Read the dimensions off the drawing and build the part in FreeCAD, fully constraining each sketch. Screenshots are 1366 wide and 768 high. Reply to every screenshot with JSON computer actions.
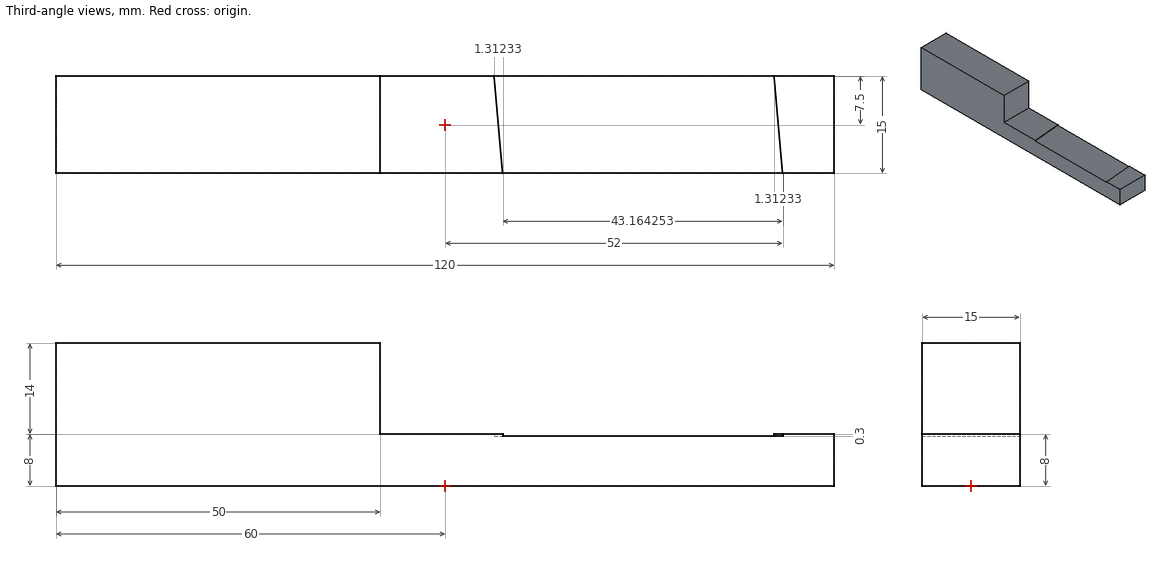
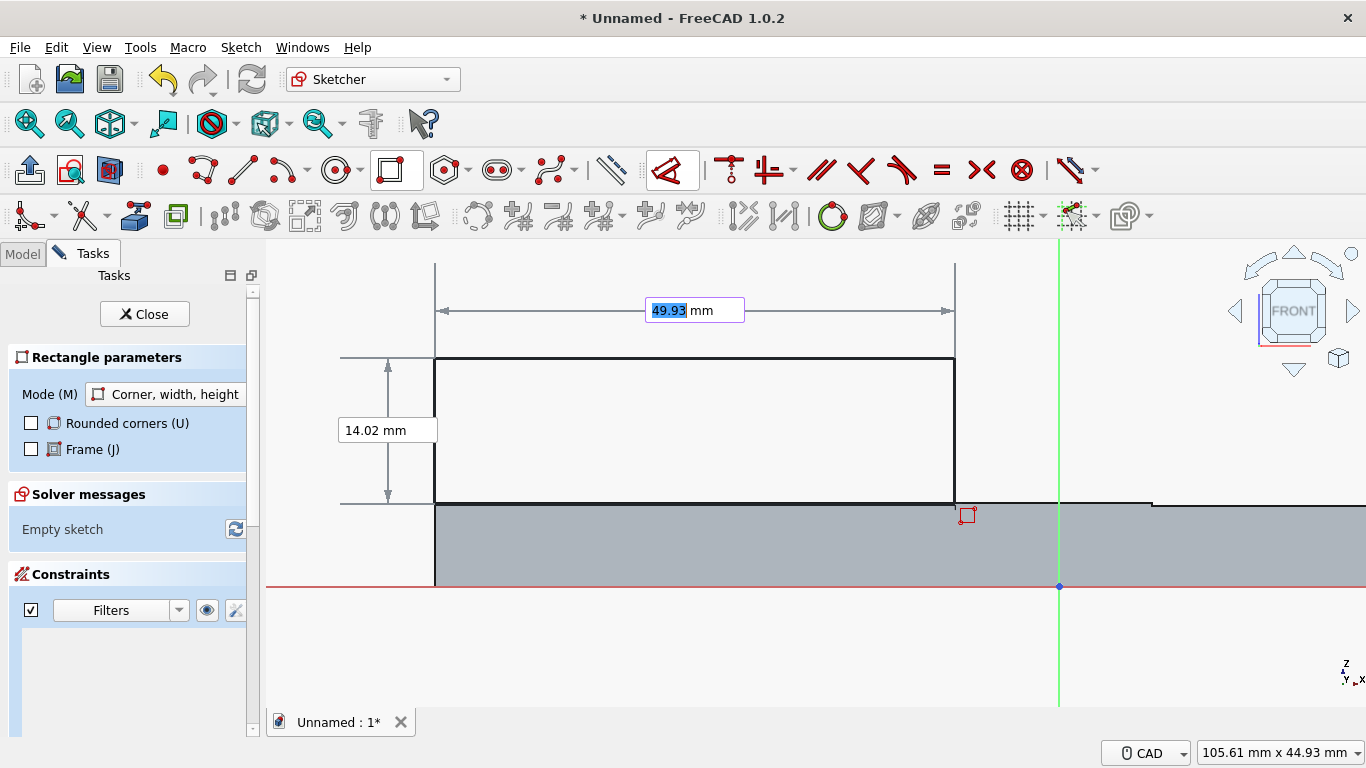
{"action": "type", "text": "50"}
{"action": "key", "text": "Tab"}
{"action": "type", "text": "14"}
{"action": "key", "text": "Return"}
{"action": "key", "text": "Escape"}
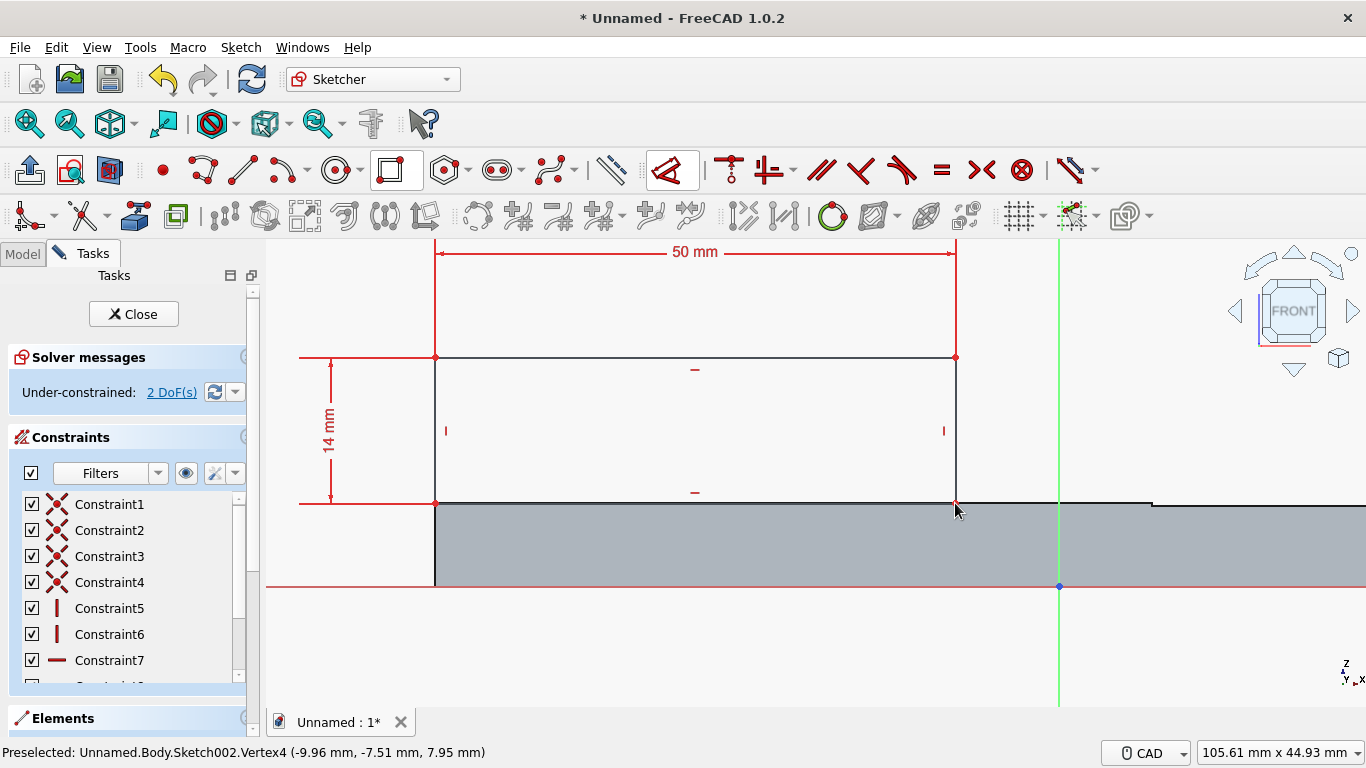
{"action": "left_click", "coordinate": [435, 504]}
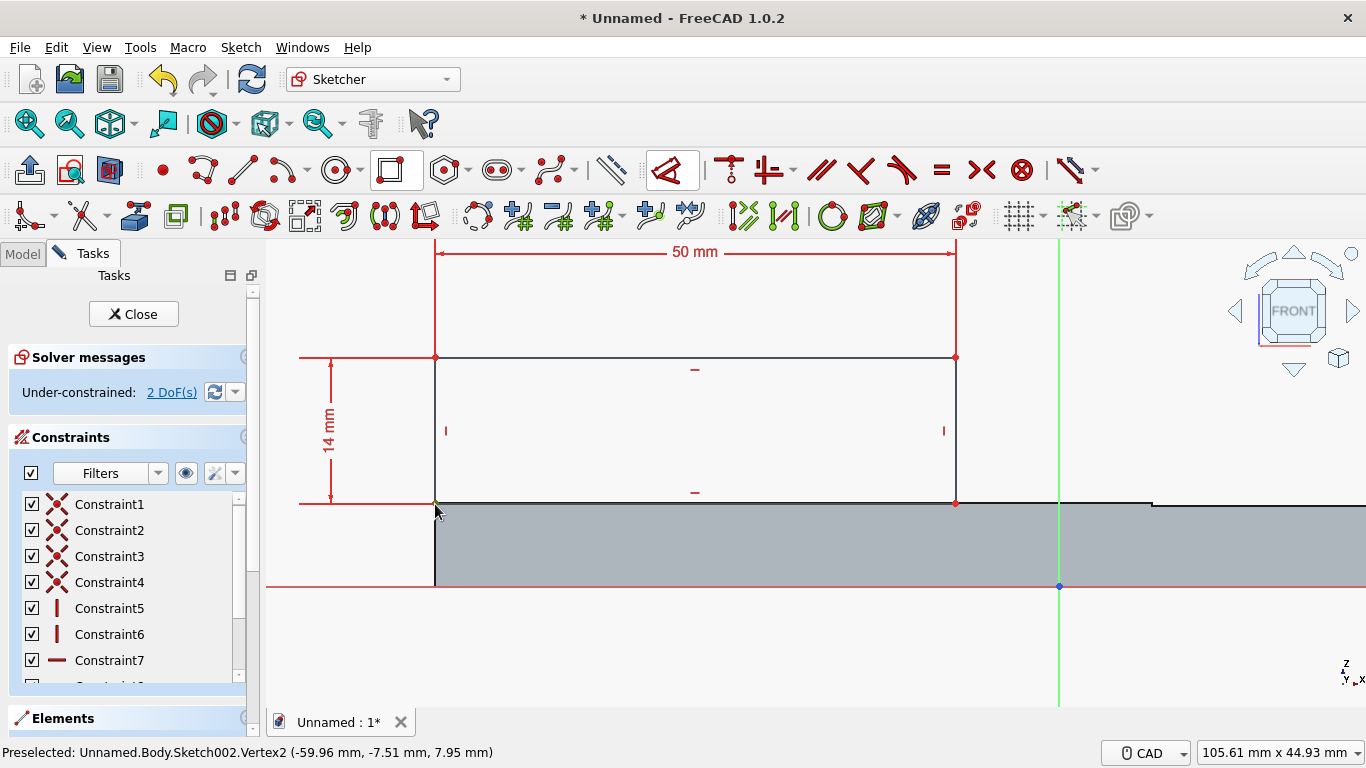
{"action": "key", "text": "i"}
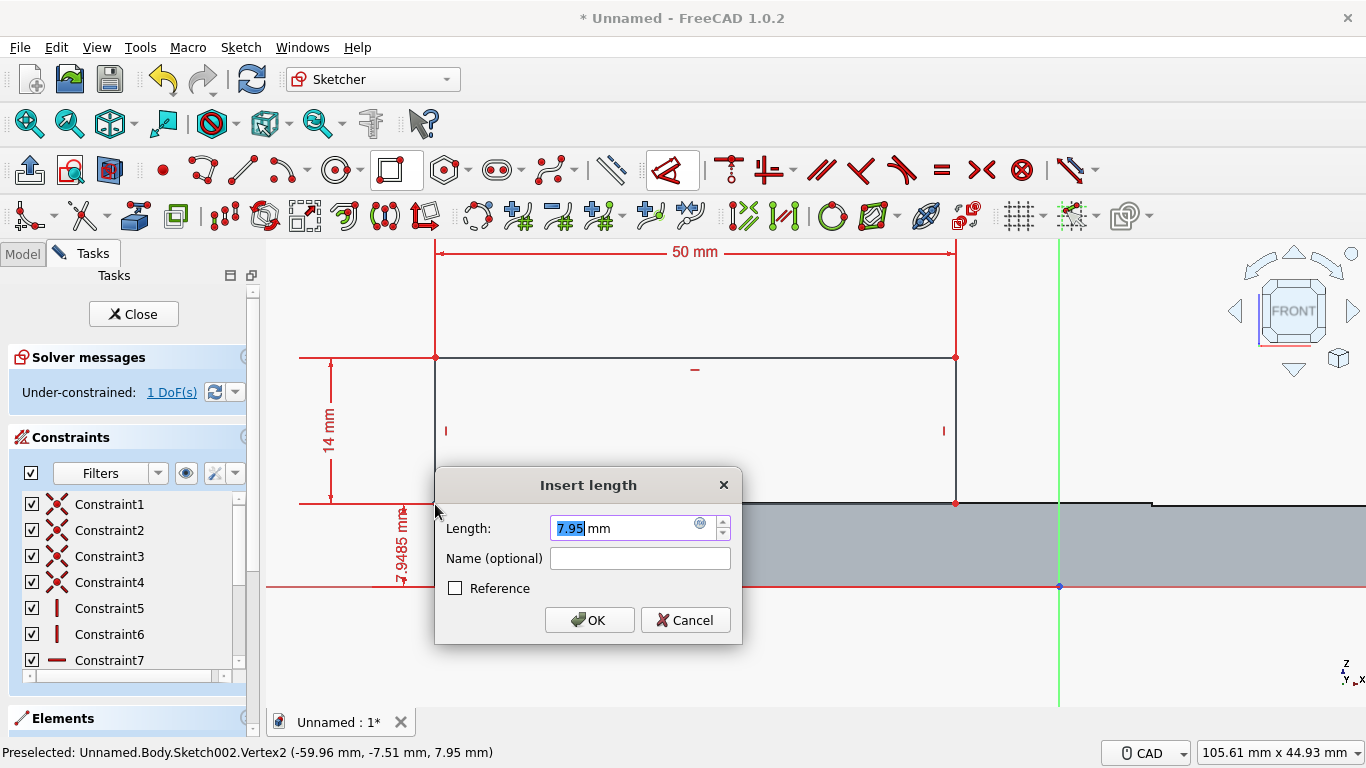
{"action": "type", "text": "8"}
{"action": "key", "text": "Return"}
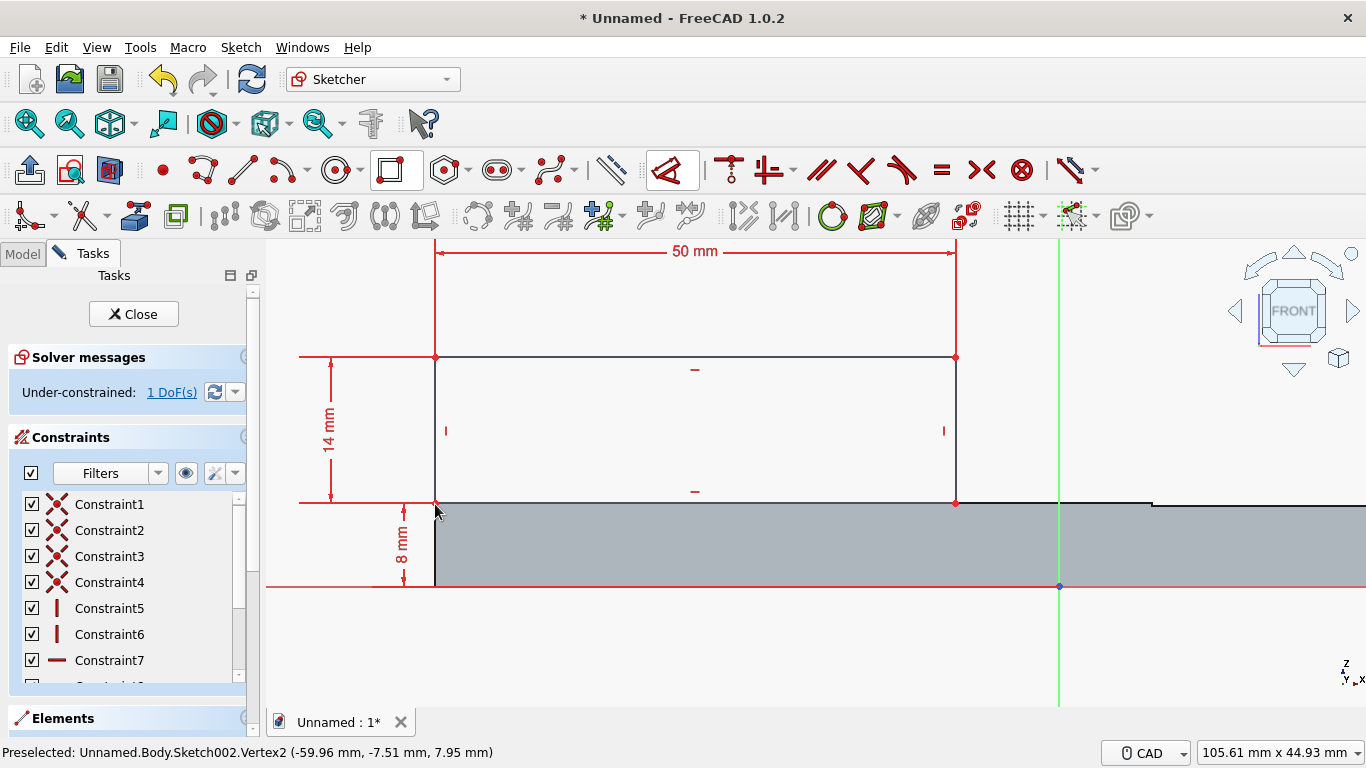
{"action": "left_click", "coordinate": [435, 357]}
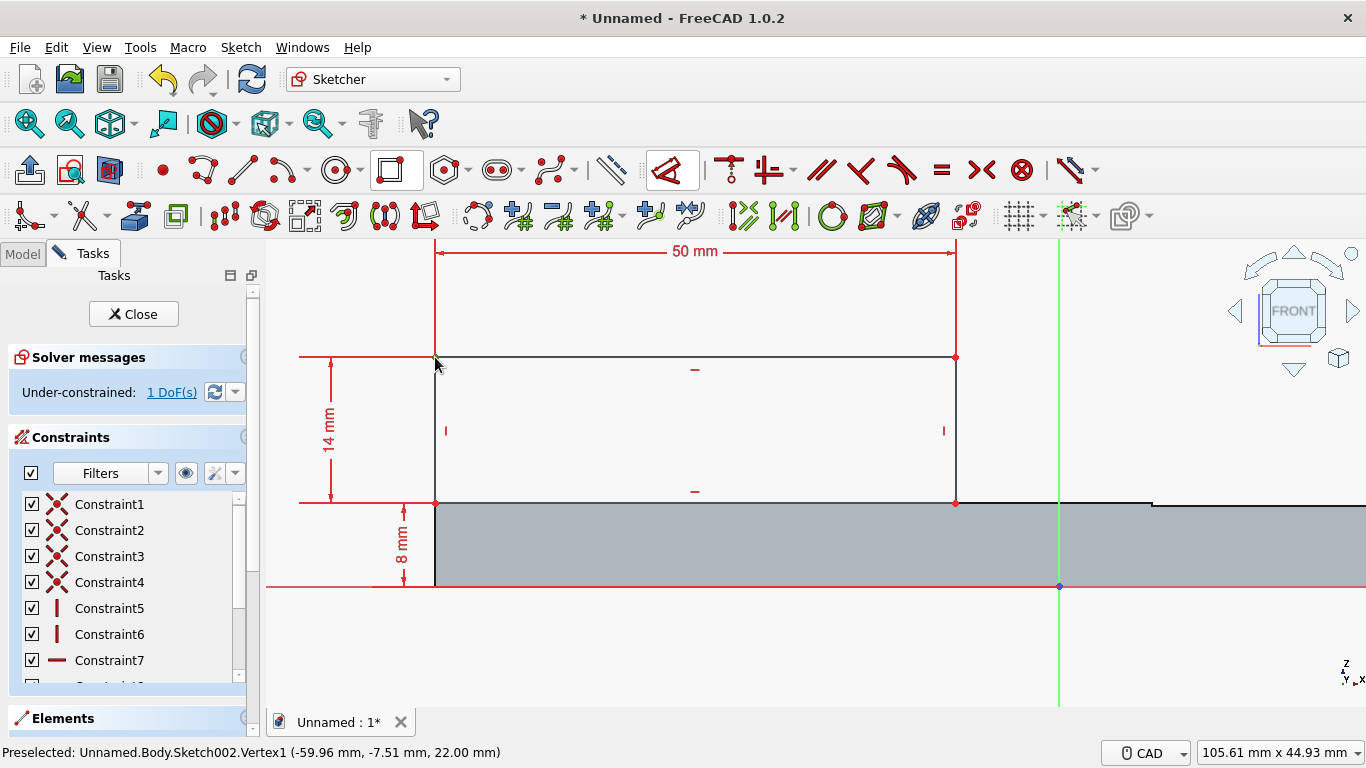
{"action": "left_click", "coordinate": [694, 170]}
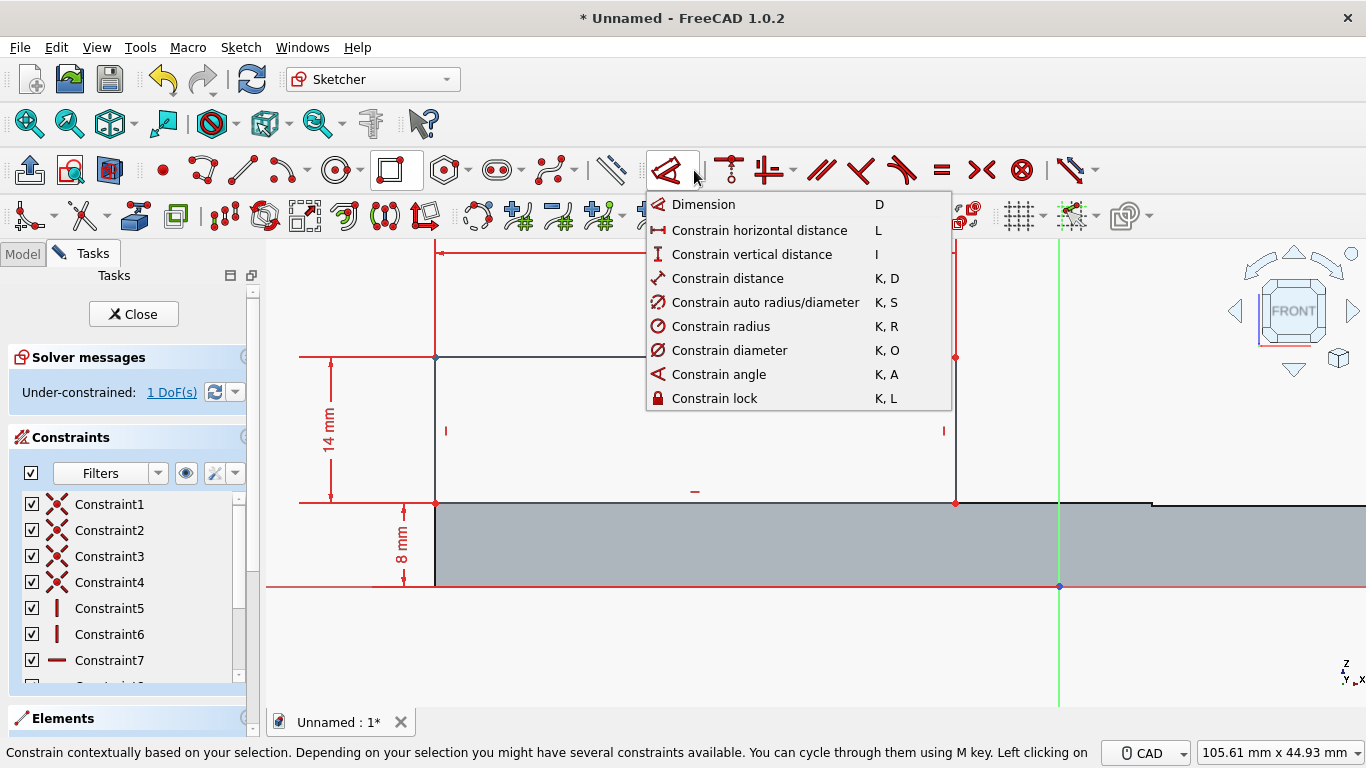
{"action": "left_click", "coordinate": [799, 230]}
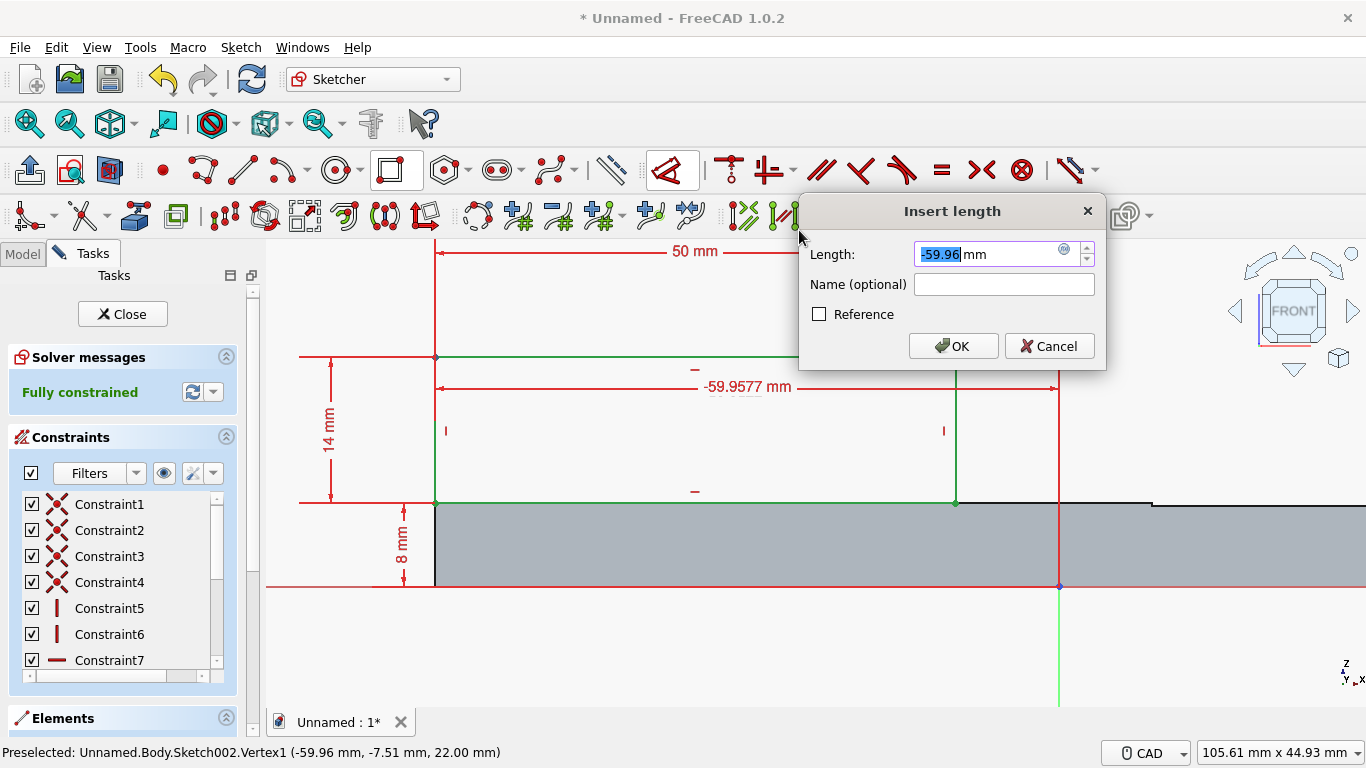
{"action": "type", "text": "-60"}
{"action": "key", "text": "Return"}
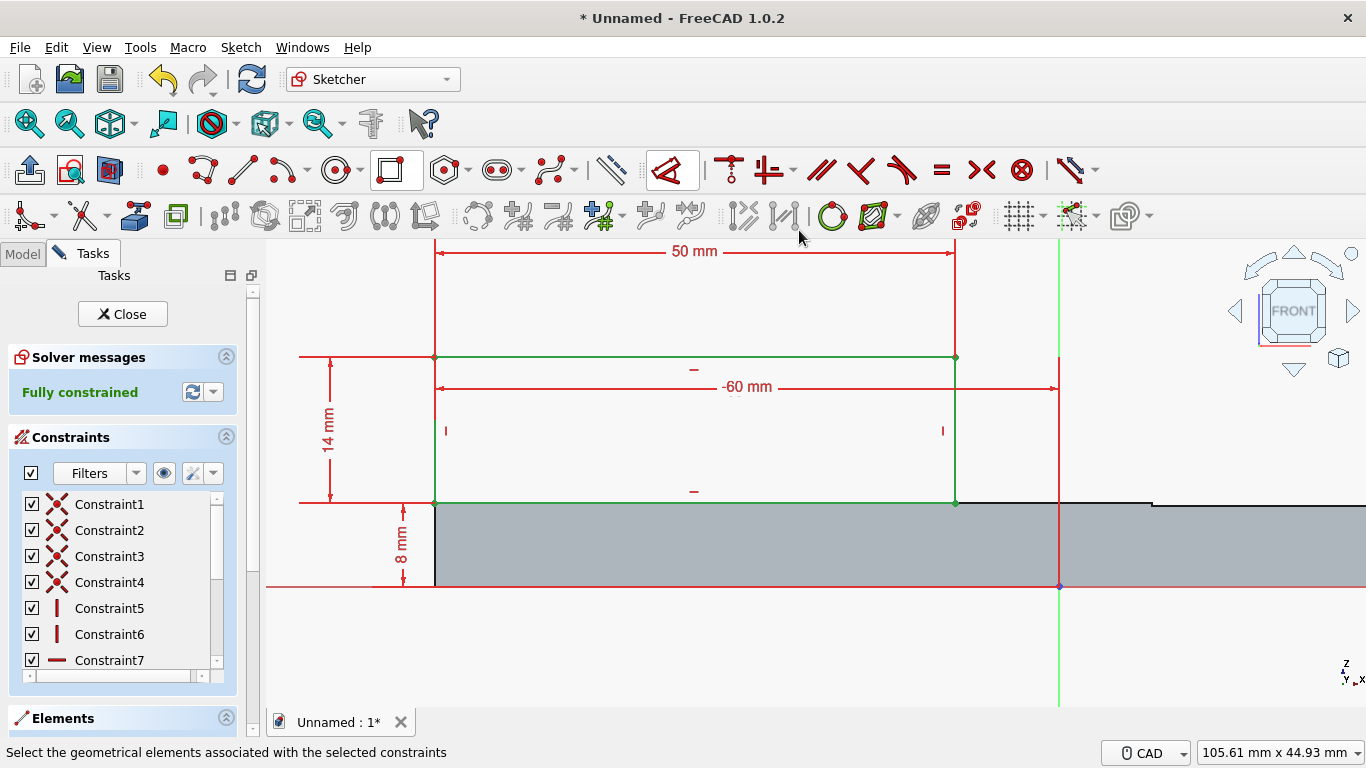
{"action": "left_click", "coordinate": [123, 314]}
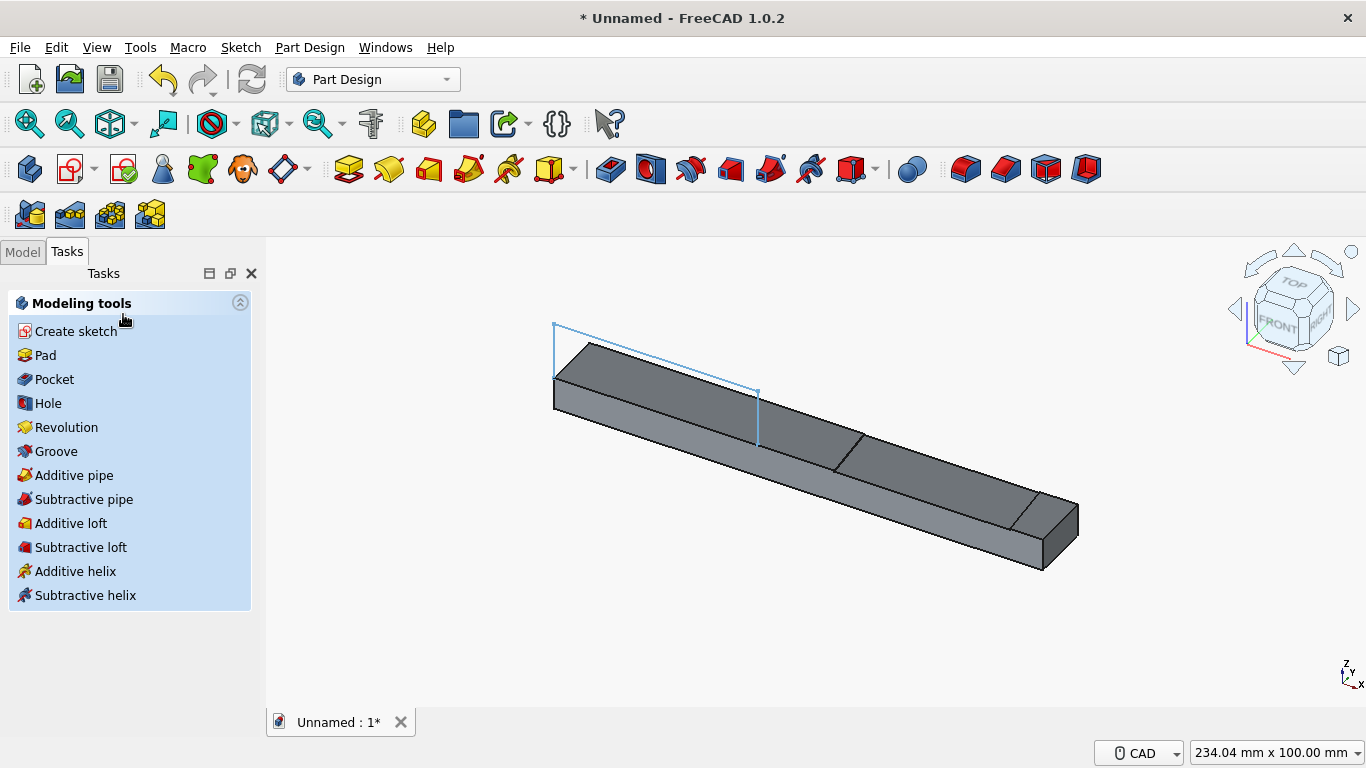
{"action": "left_click", "coordinate": [350, 170]}